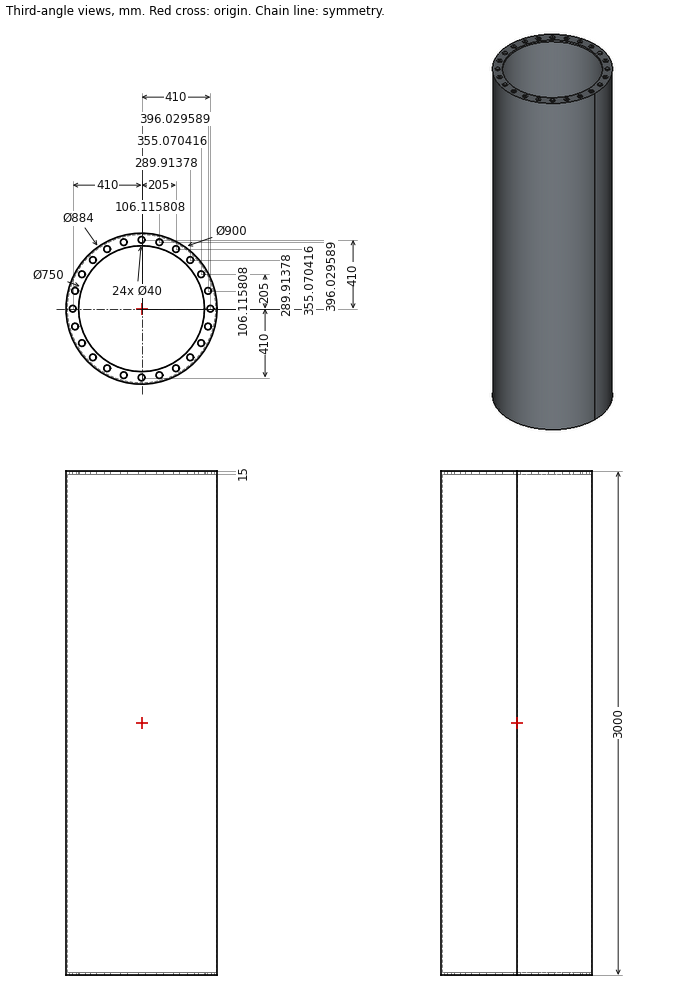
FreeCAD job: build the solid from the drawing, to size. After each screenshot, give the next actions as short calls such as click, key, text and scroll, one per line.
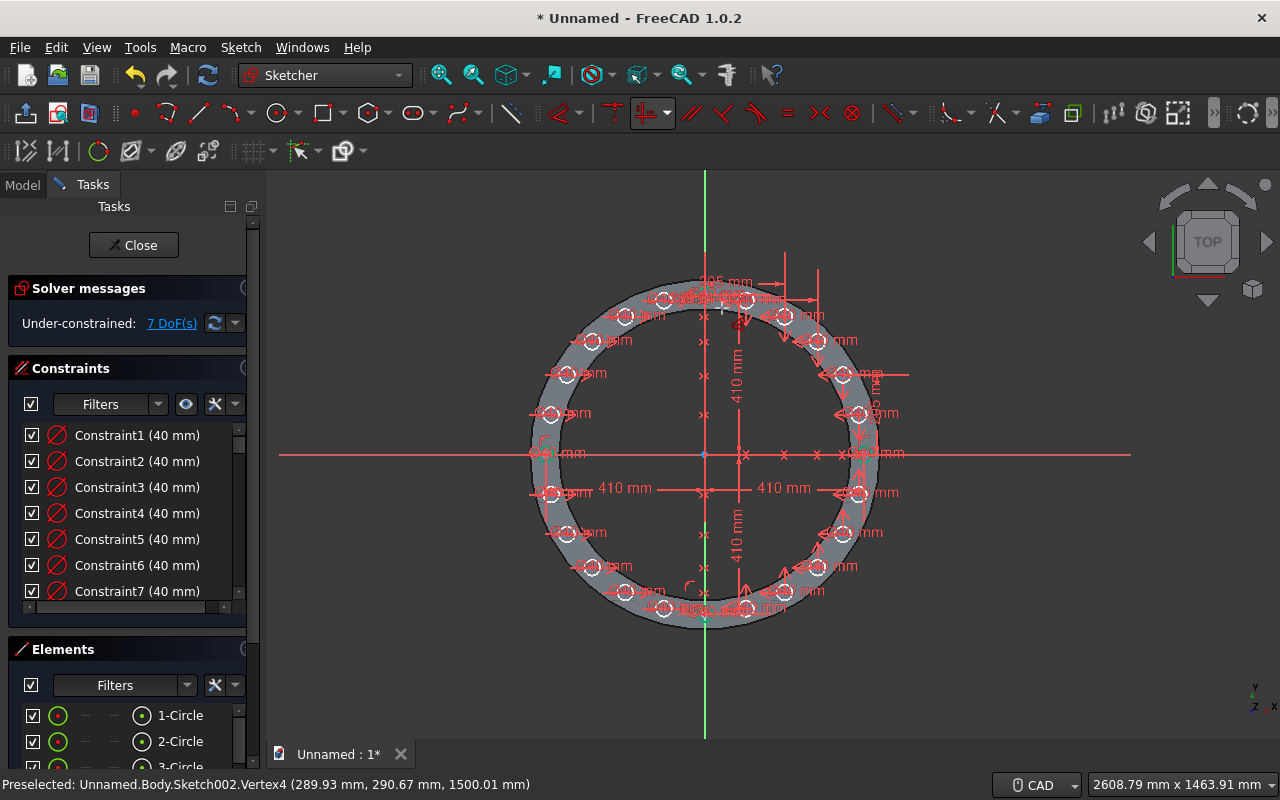
click(818, 342)
click(852, 438)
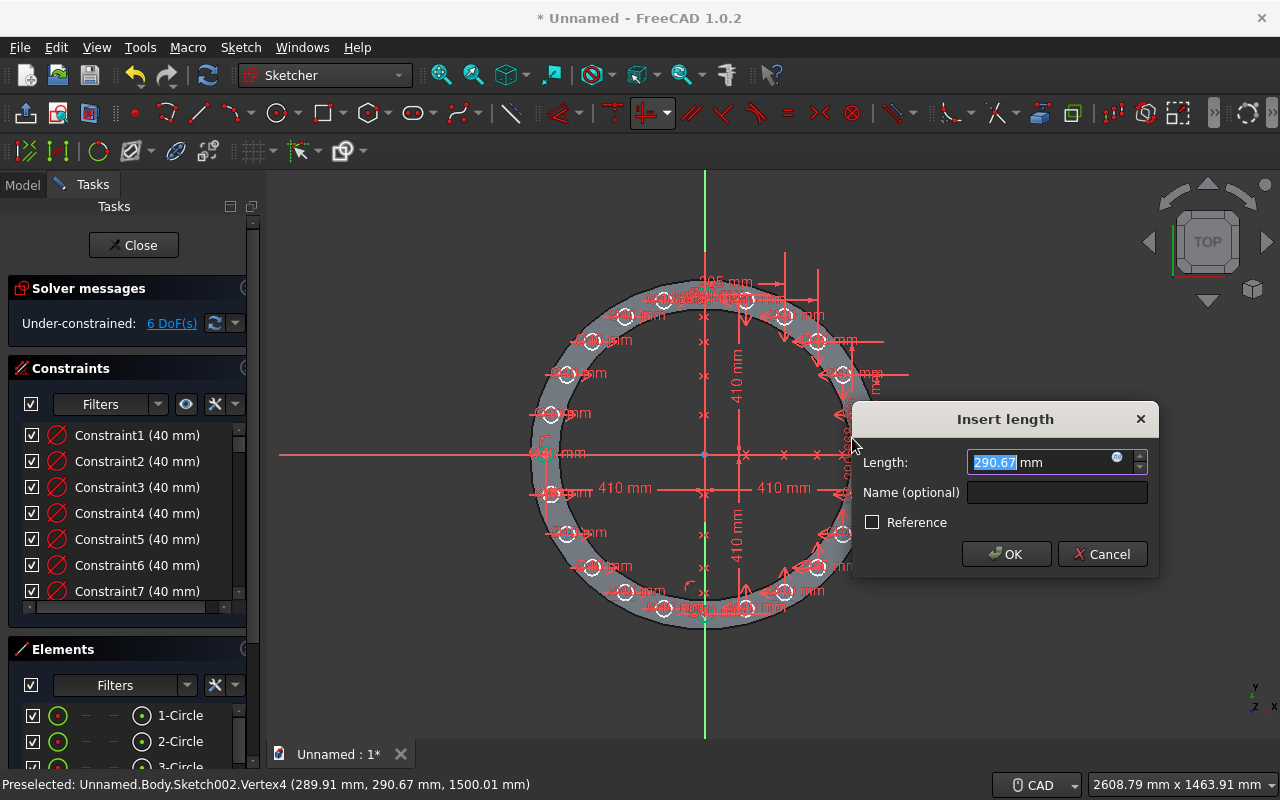
text(289.91378)
key(Return)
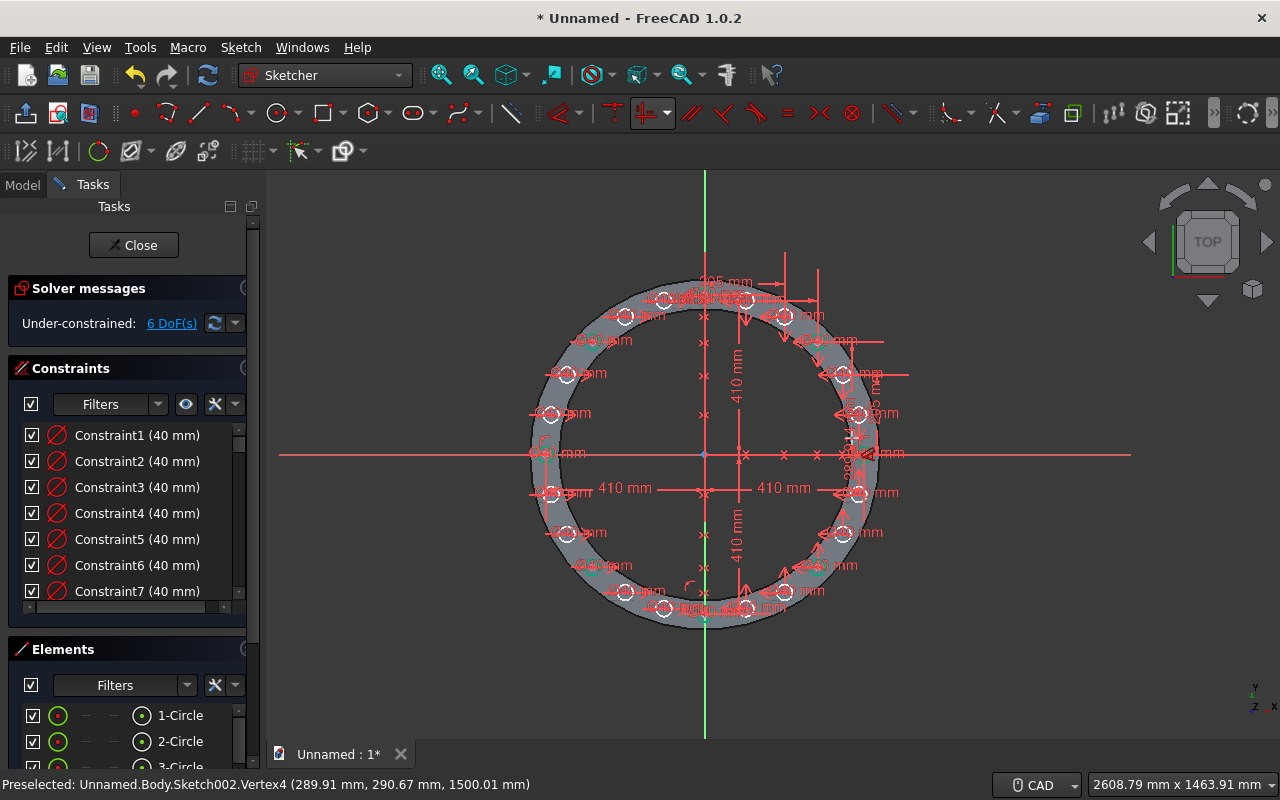
click(746, 301)
click(725, 243)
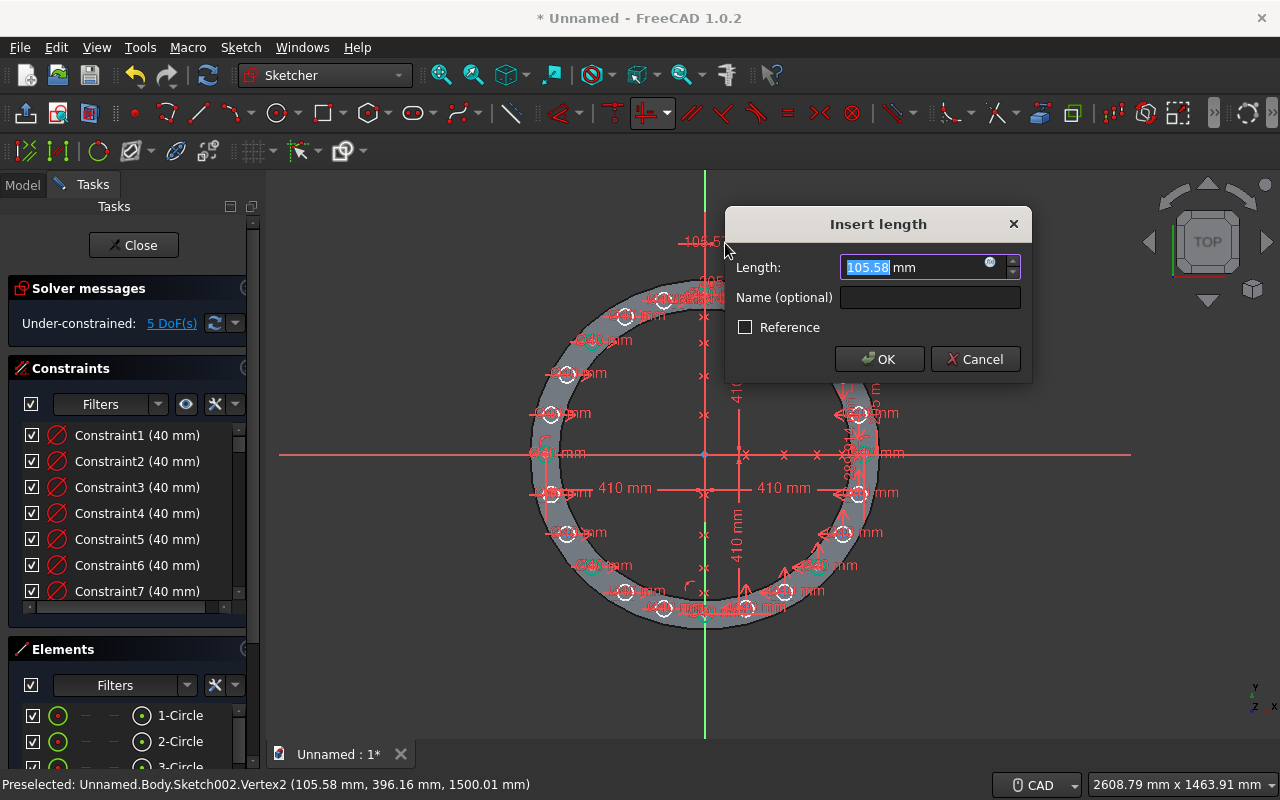
text(106.115808)
key(Return)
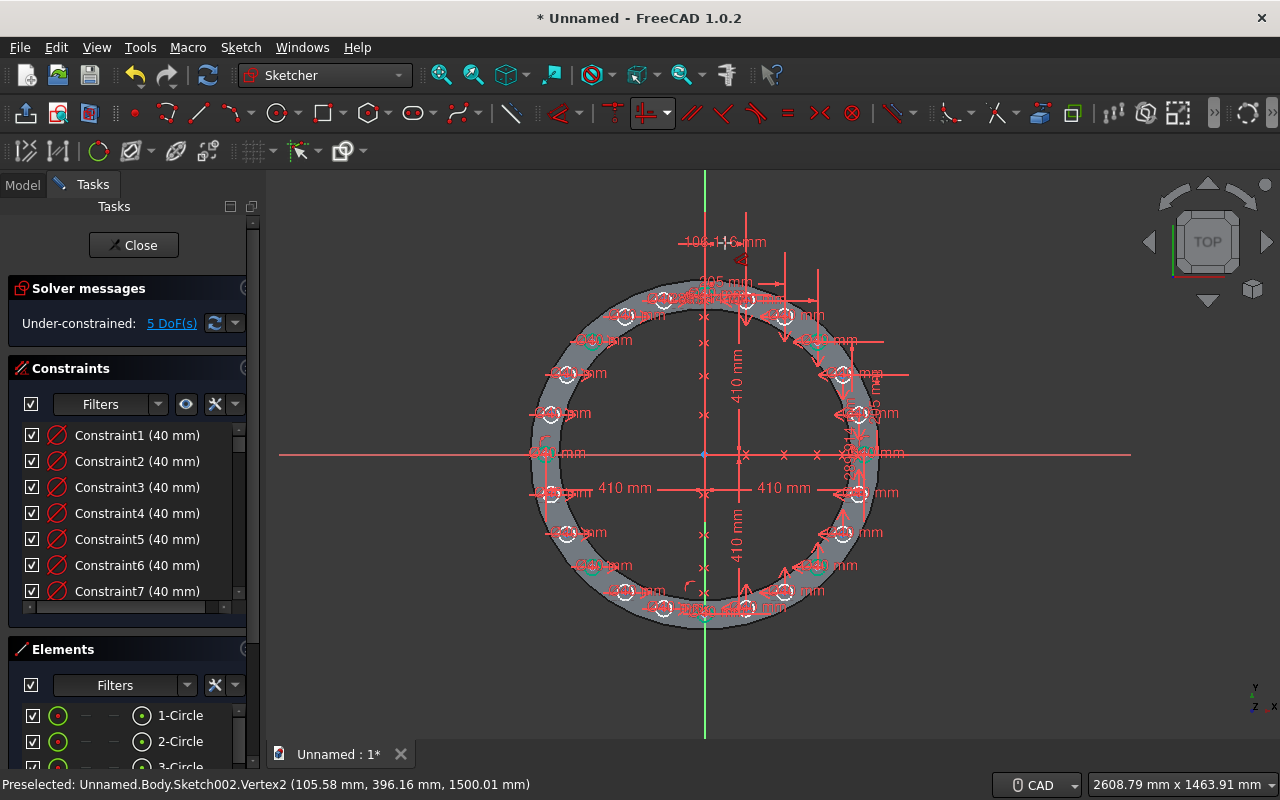
click(746, 301)
click(780, 342)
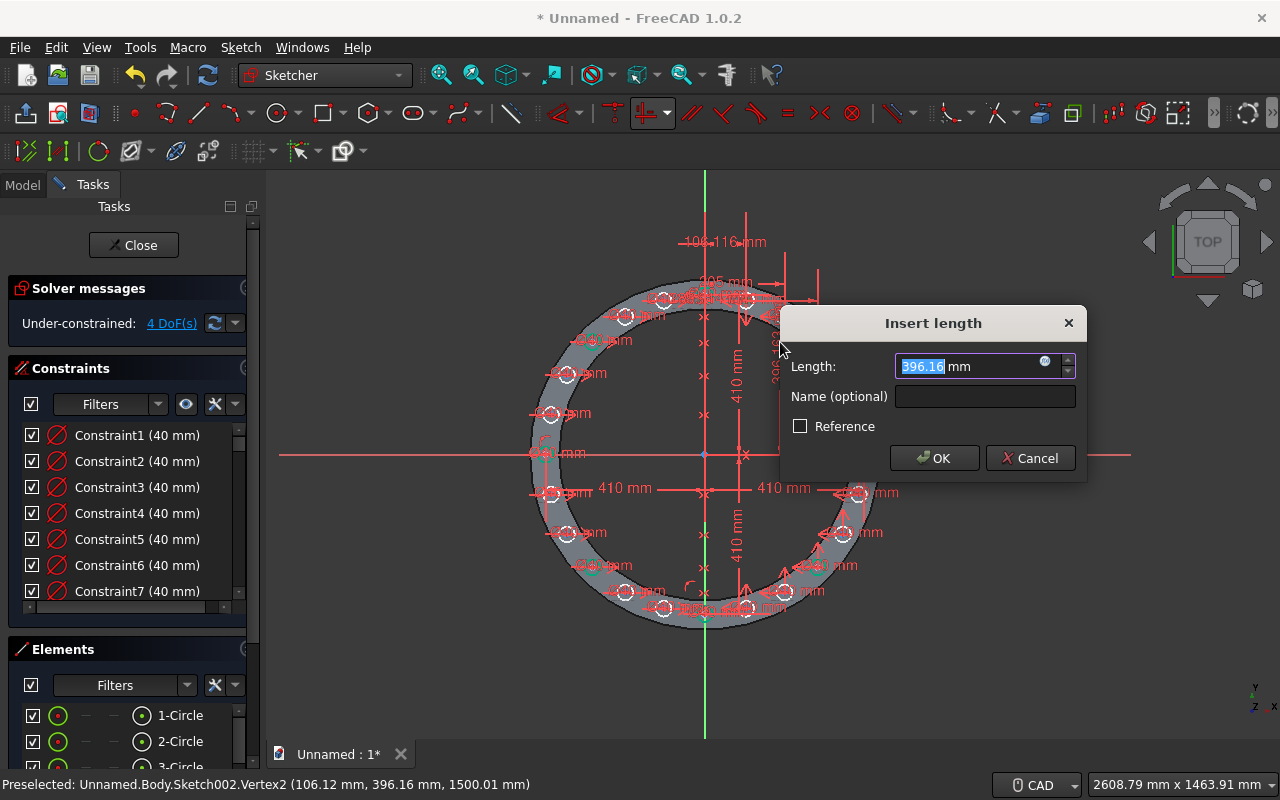
text(396.029589)
key(Return)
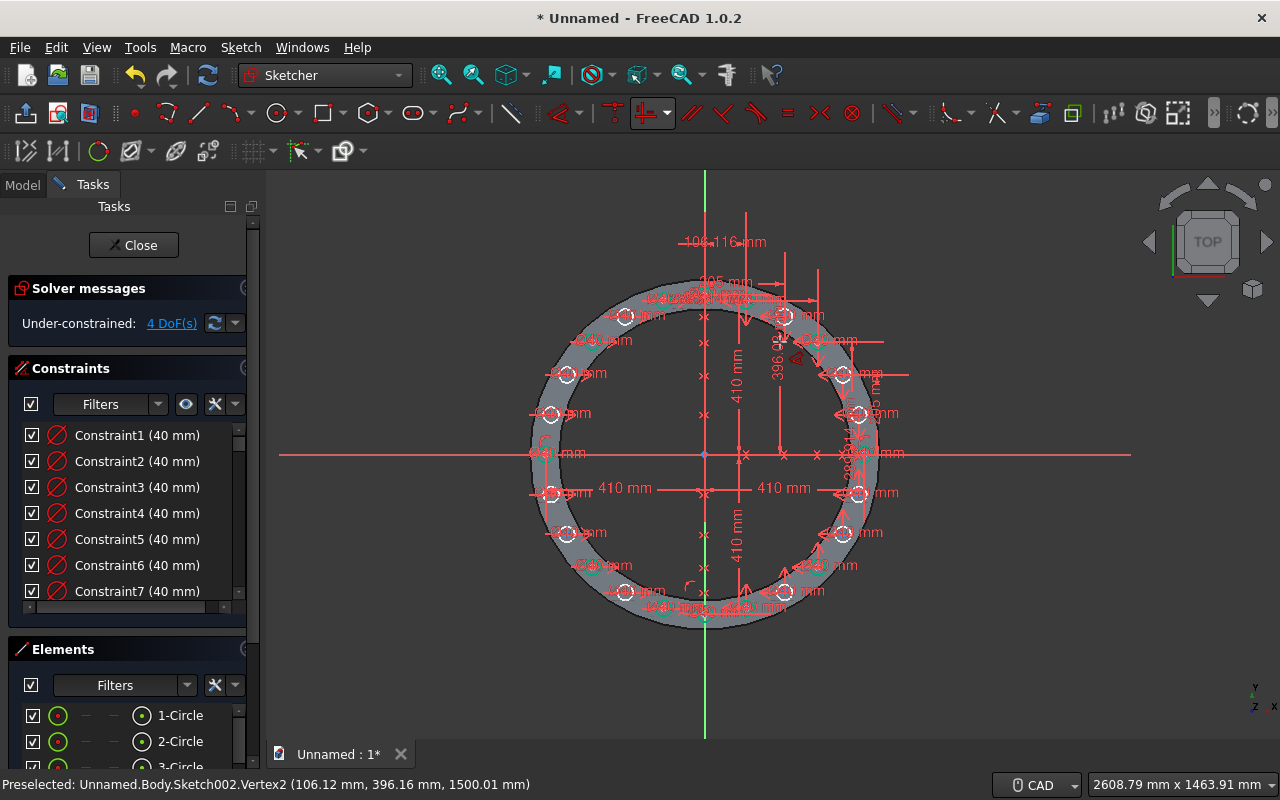
click(785, 317)
click(819, 418)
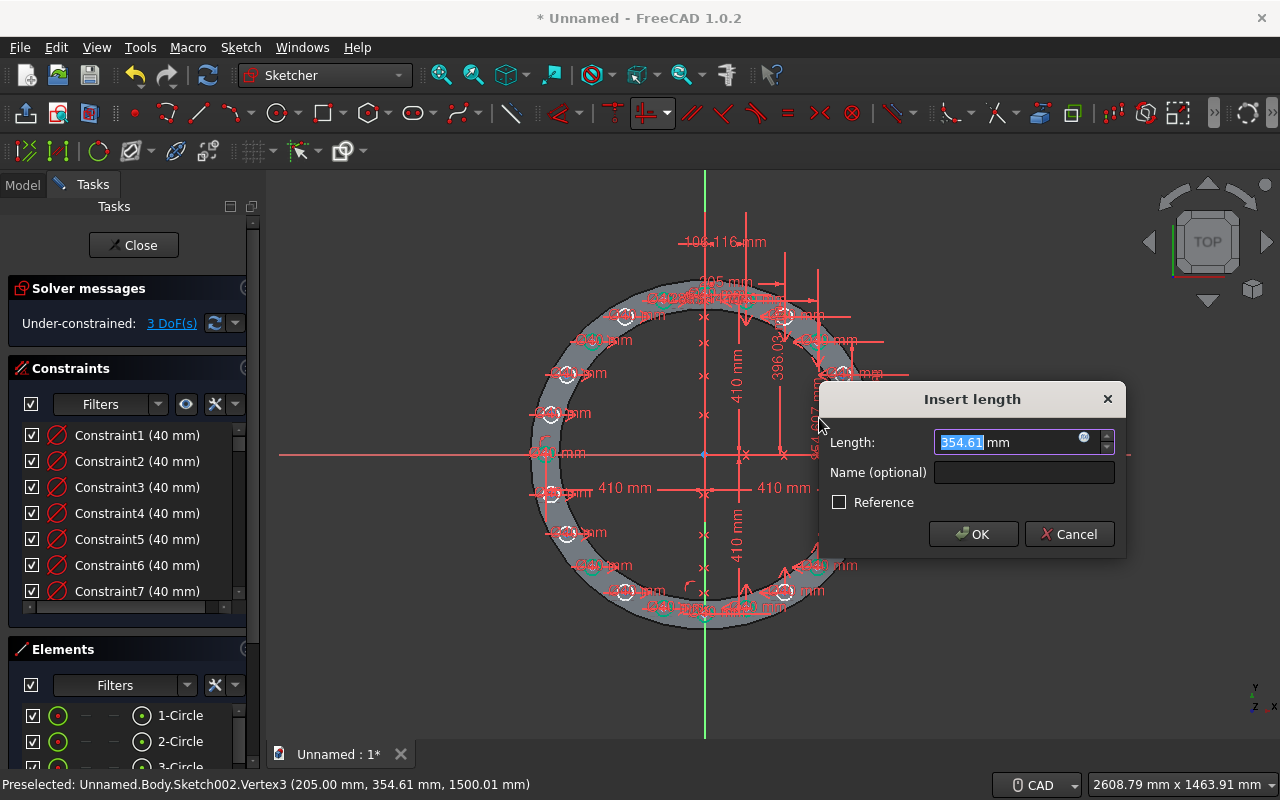
text(355.070416)
key(Return)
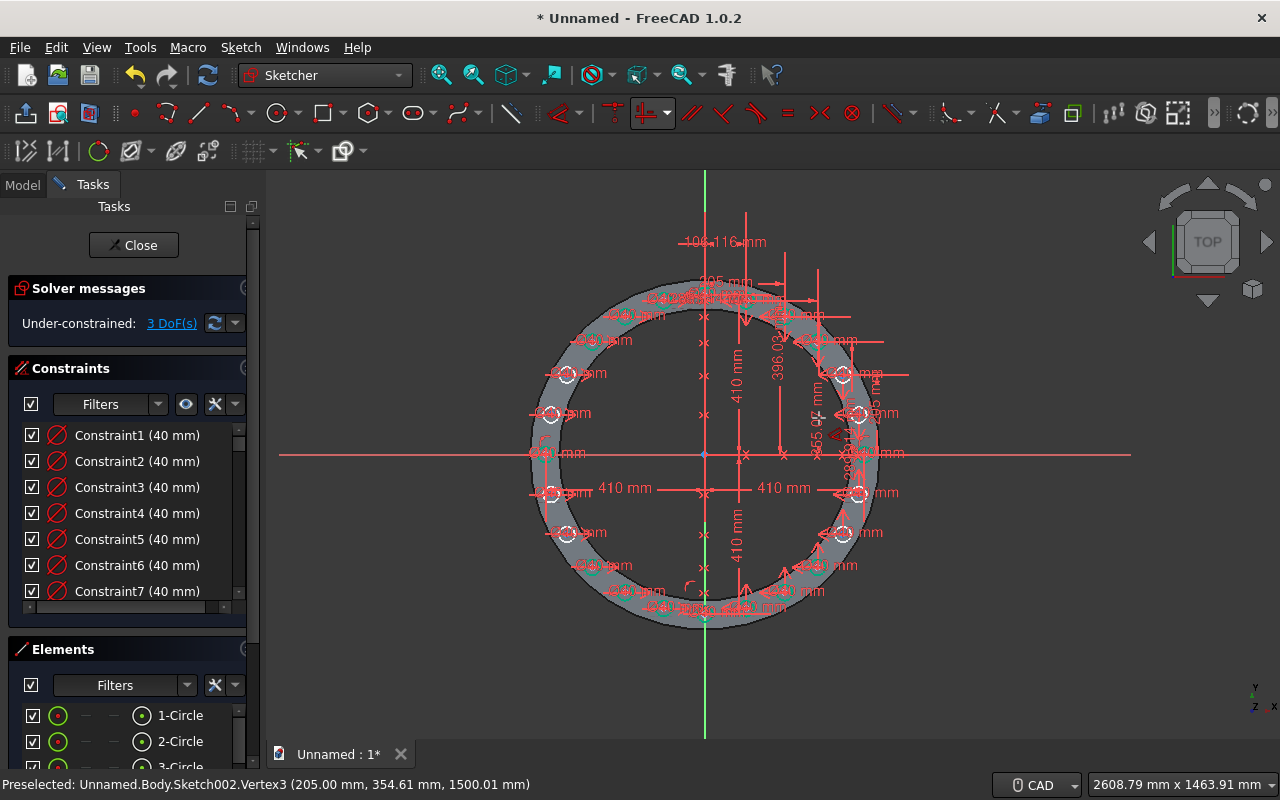
click(843, 375)
click(806, 317)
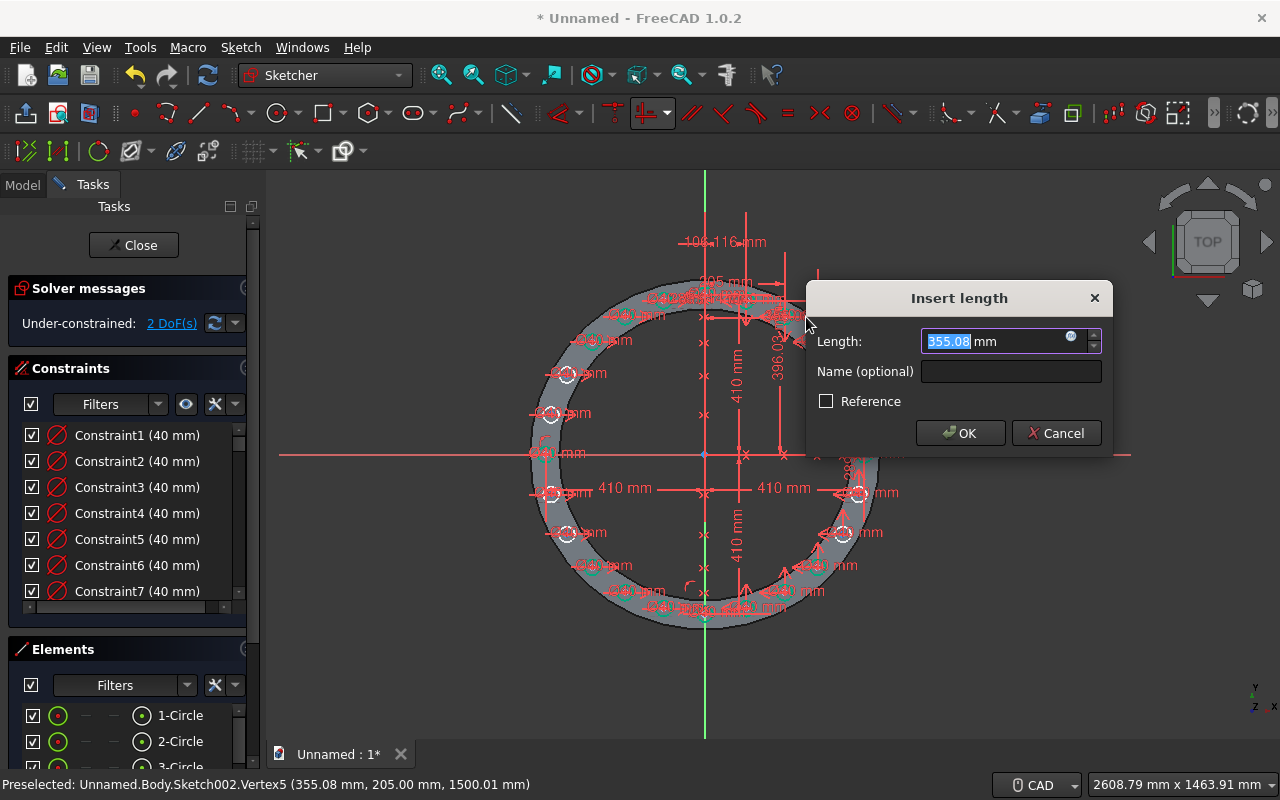
text(355.070416)
key(Return)